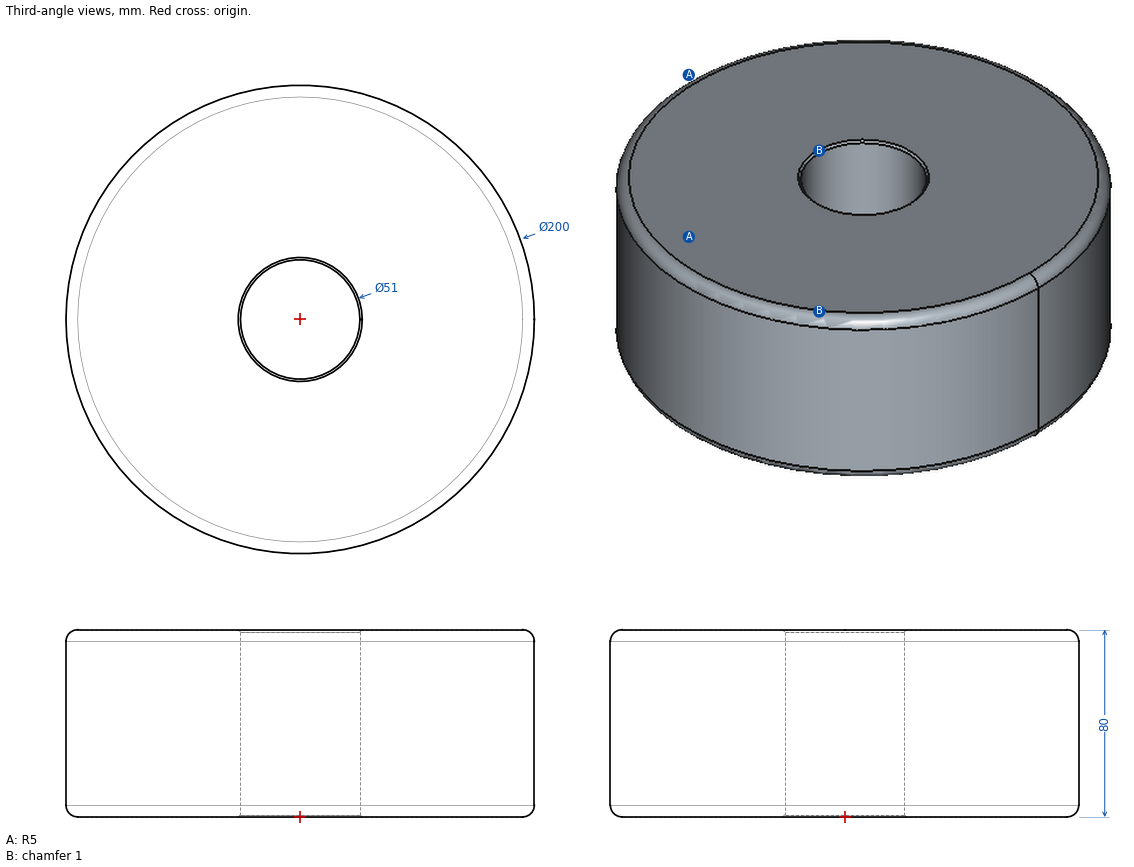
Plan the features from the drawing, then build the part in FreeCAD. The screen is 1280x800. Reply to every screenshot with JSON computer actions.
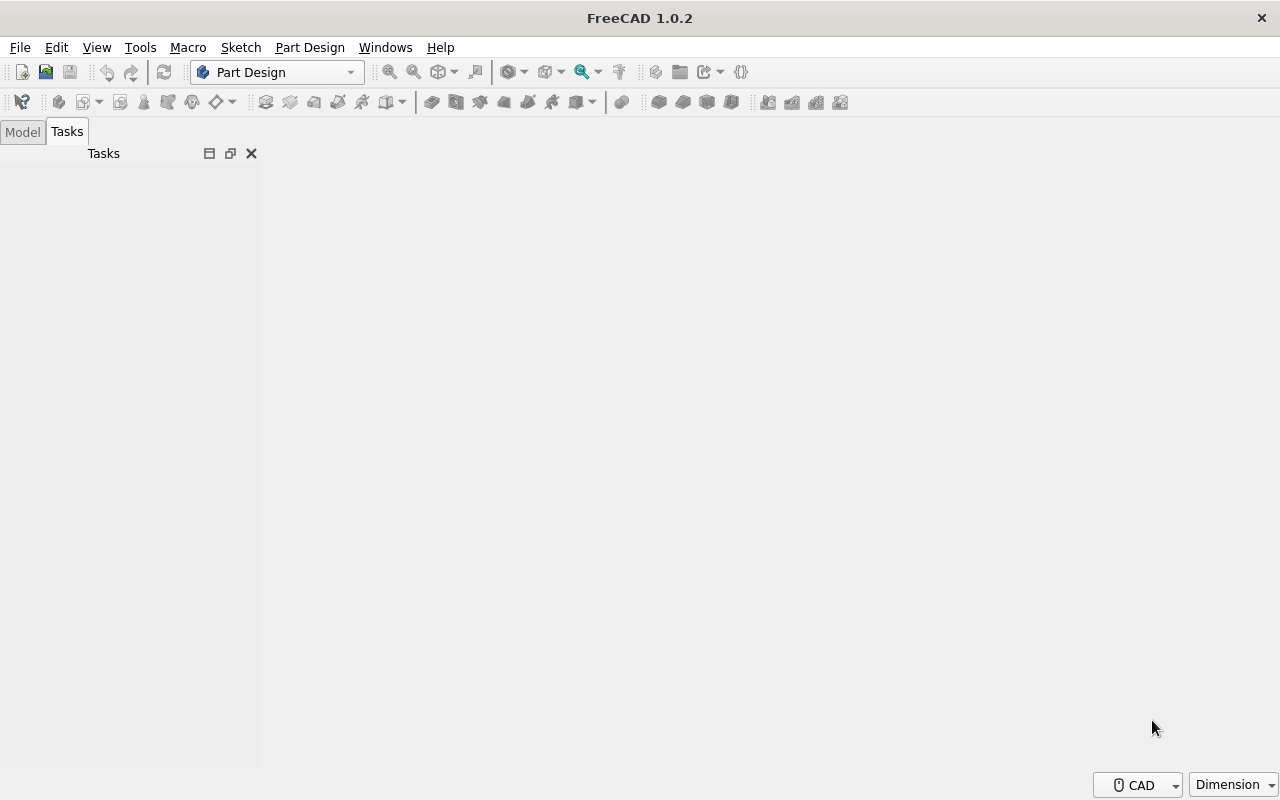
{"action": "left_click", "coordinate": [22, 72]}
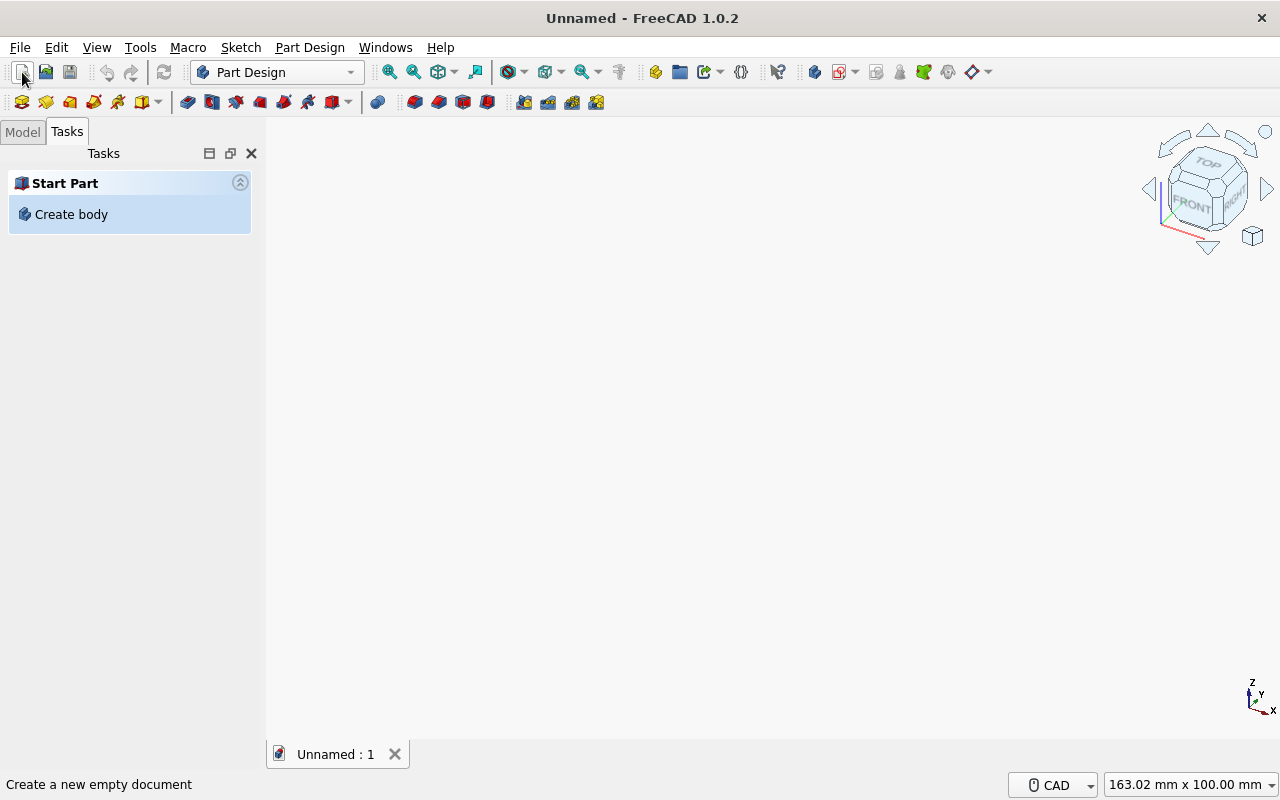
{"action": "left_click", "coordinate": [840, 72]}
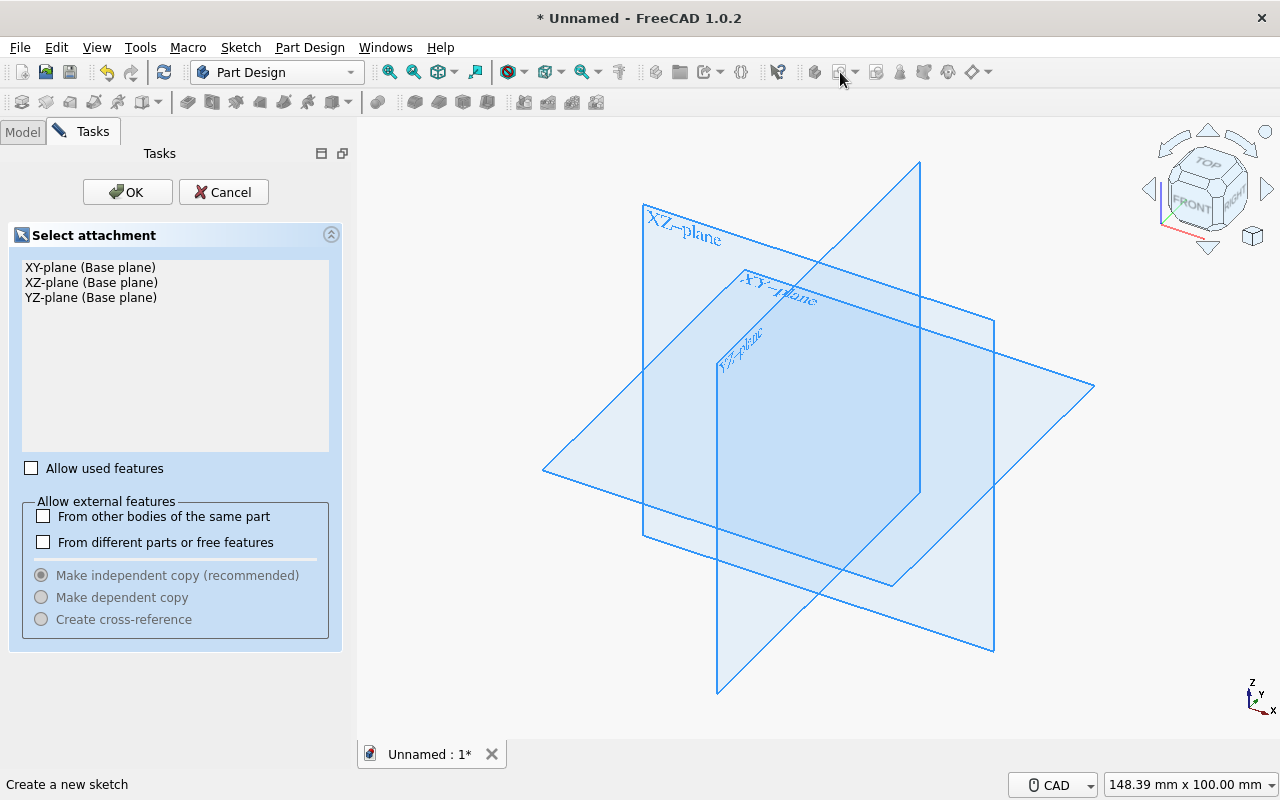
{"action": "left_click", "coordinate": [82, 268]}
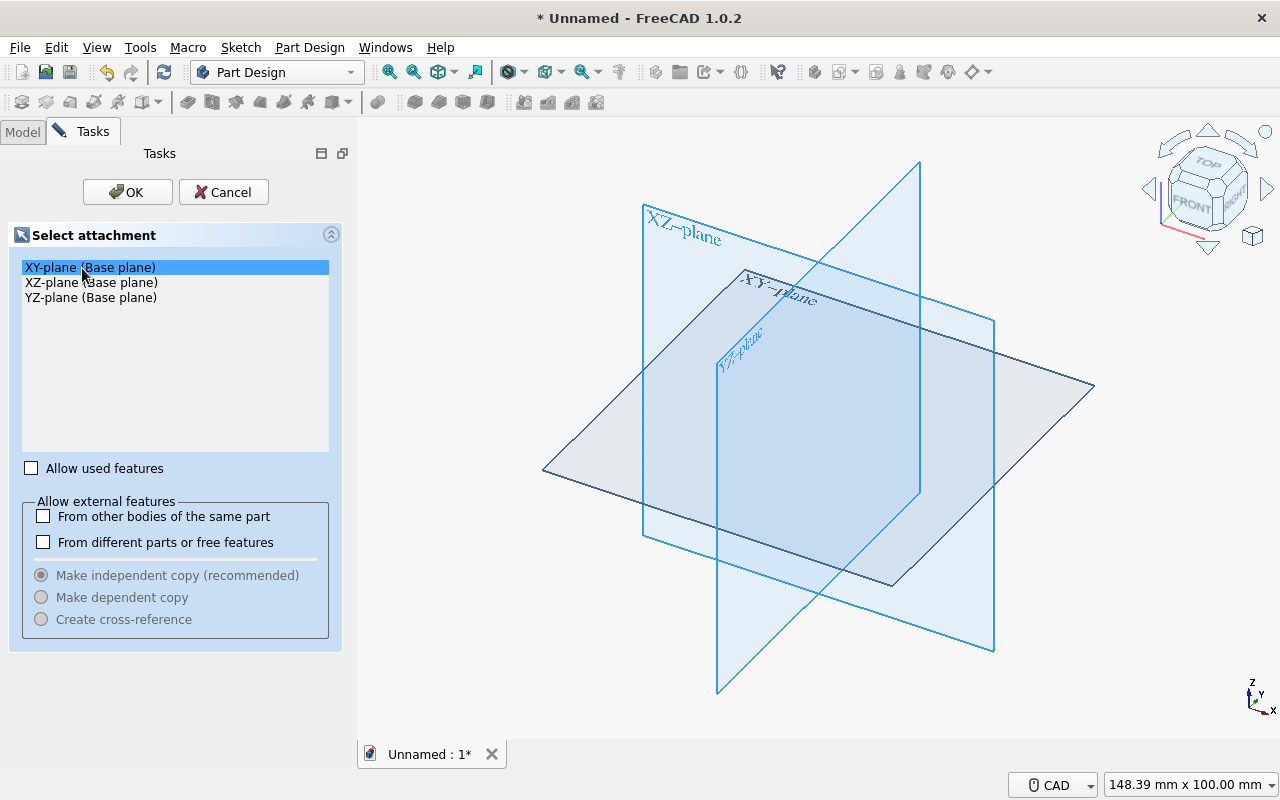
{"action": "left_click", "coordinate": [128, 192]}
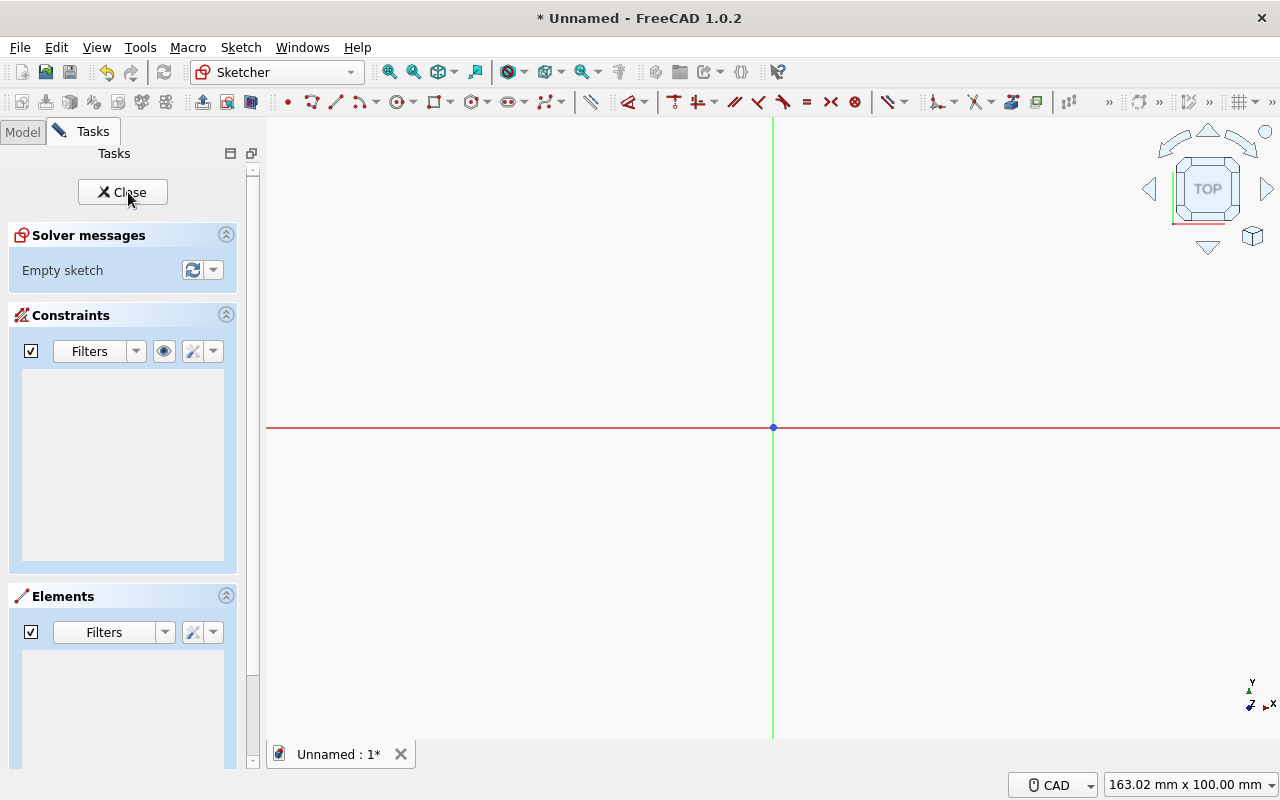
{"action": "scroll", "coordinate": [675, 428], "scroll_direction": "down", "scroll_amount": 6}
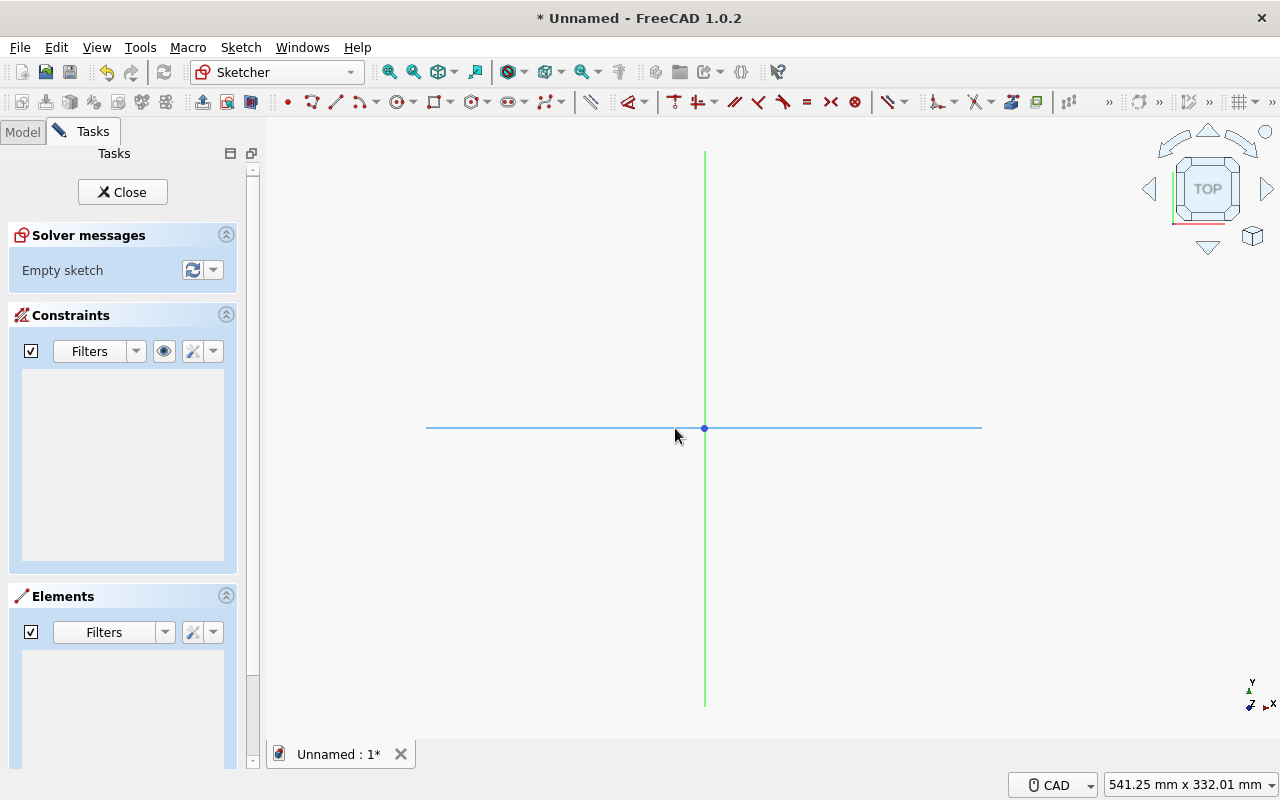
{"action": "left_click", "coordinate": [398, 102]}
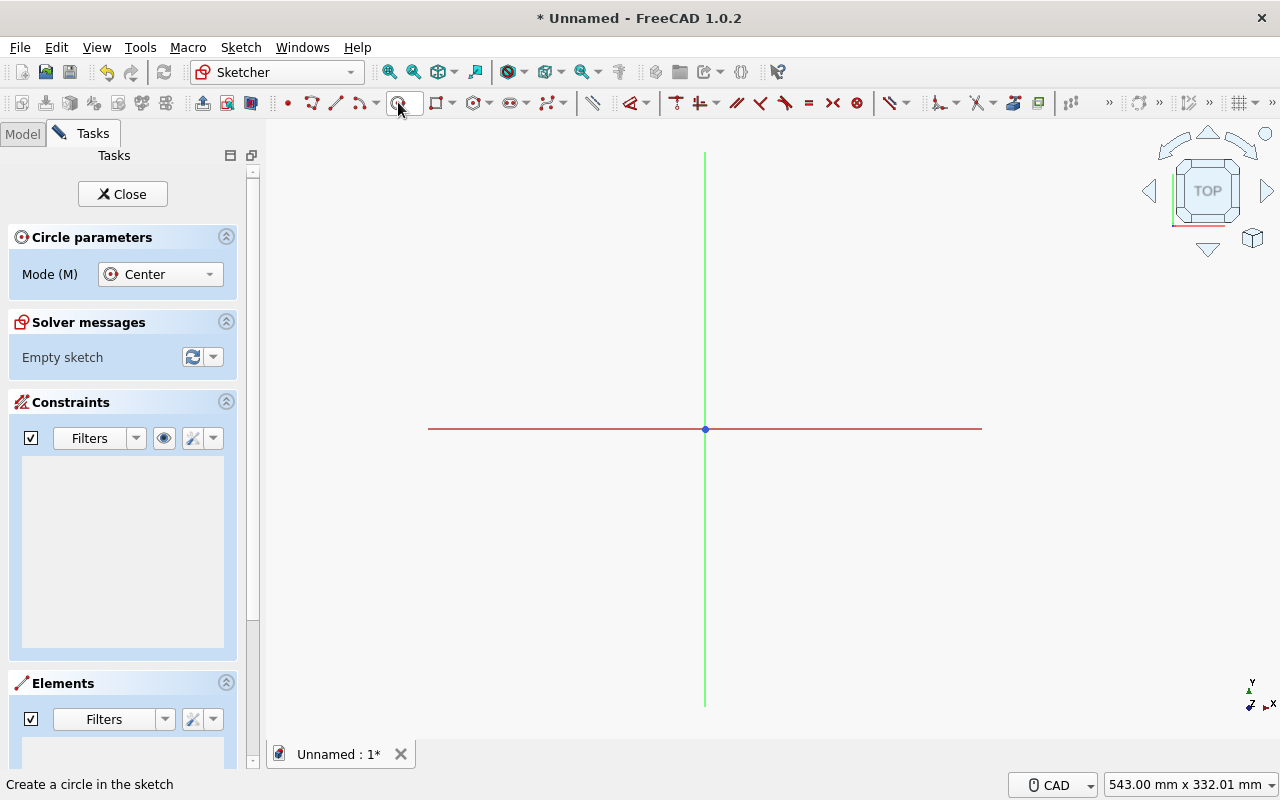
{"action": "left_click", "coordinate": [705, 429]}
{"action": "mouse_move", "coordinate": [837, 297]}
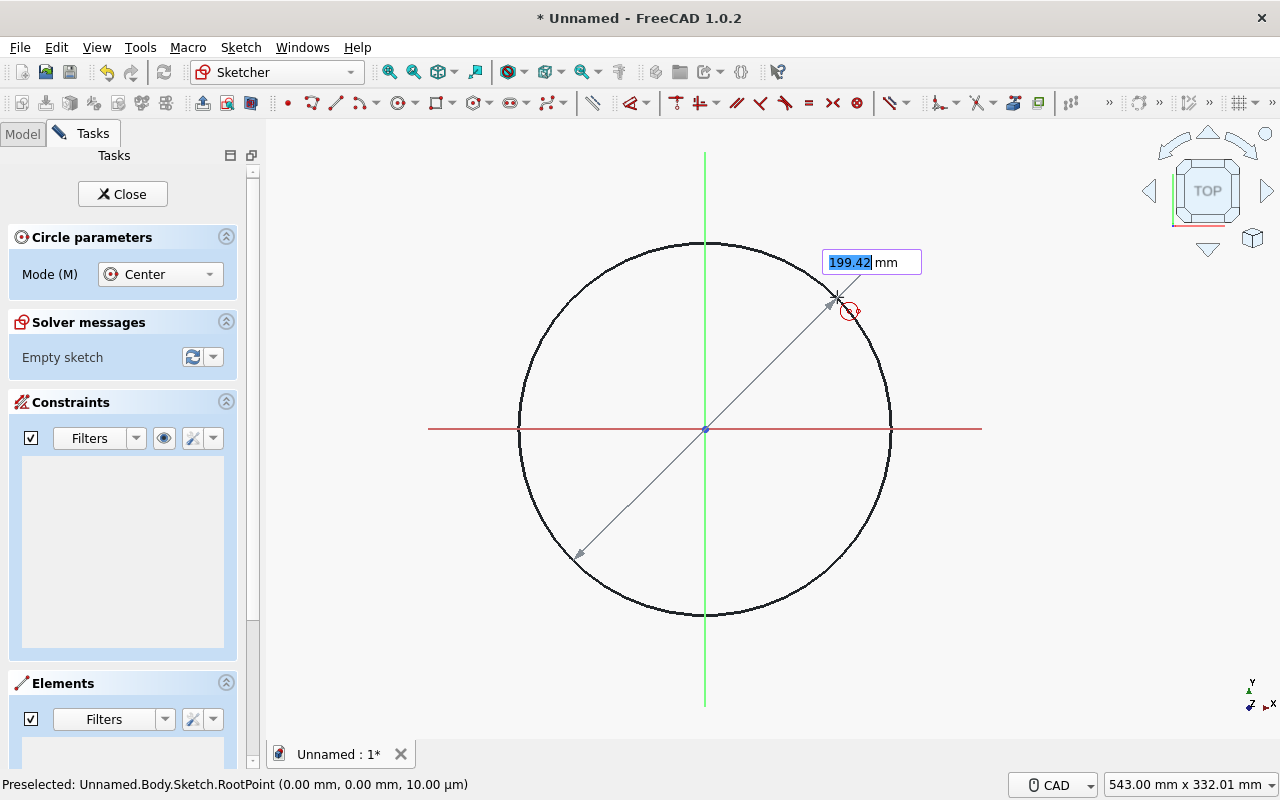
{"action": "type", "text": "200"}
{"action": "key", "text": "Return"}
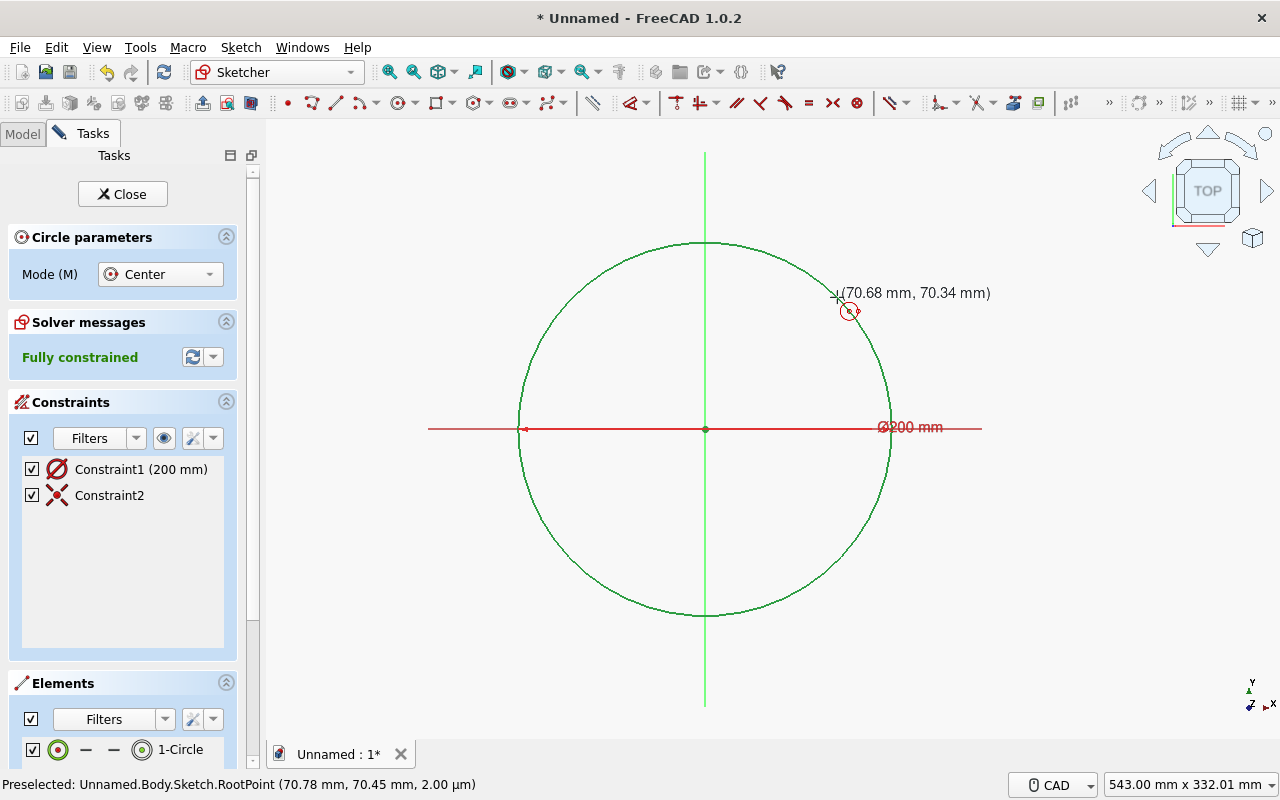
{"action": "left_click", "coordinate": [705, 429]}
{"action": "mouse_move", "coordinate": [739, 396]}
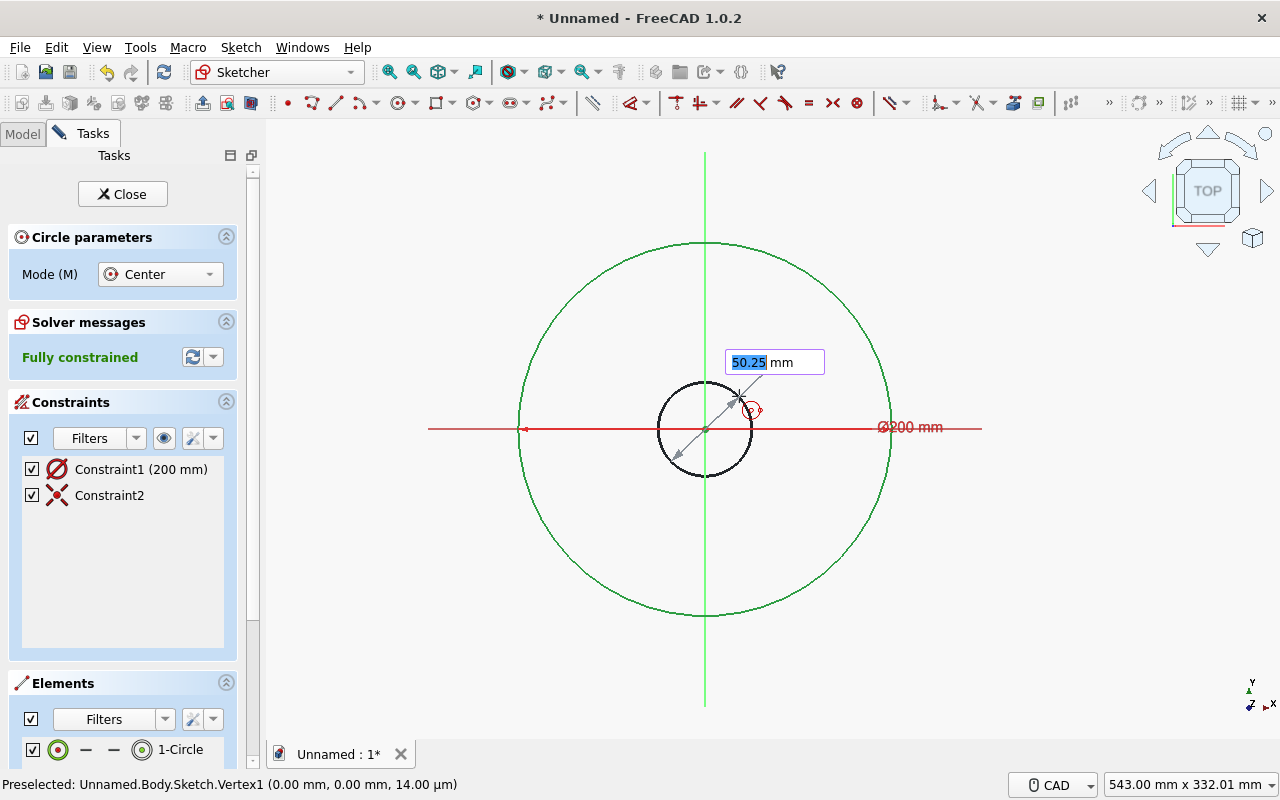
{"action": "type", "text": "51"}
{"action": "key", "text": "Return"}
{"action": "key", "text": "Escape"}